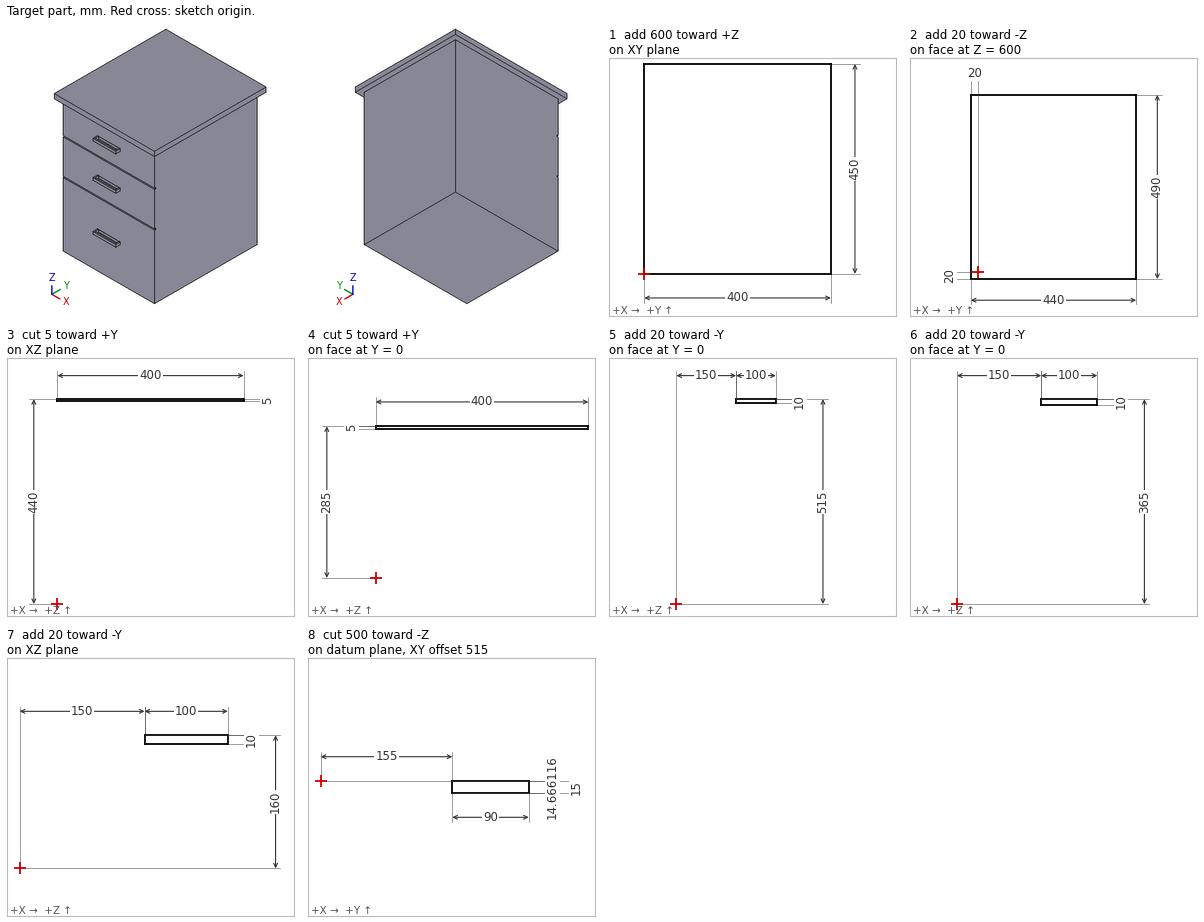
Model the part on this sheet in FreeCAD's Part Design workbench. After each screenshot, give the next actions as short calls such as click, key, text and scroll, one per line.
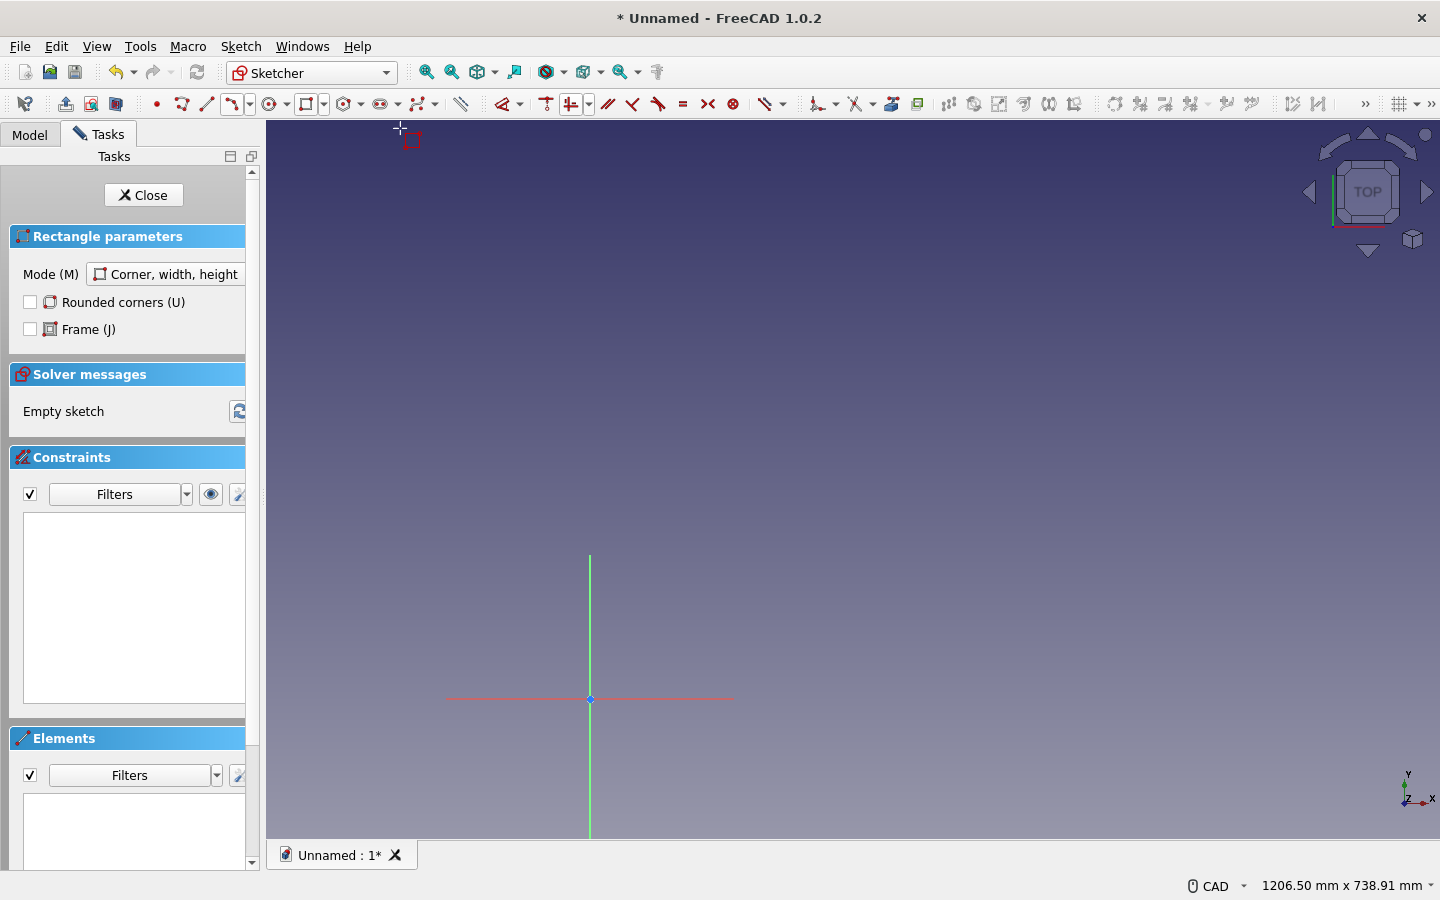
click(590, 699)
move(980, 262)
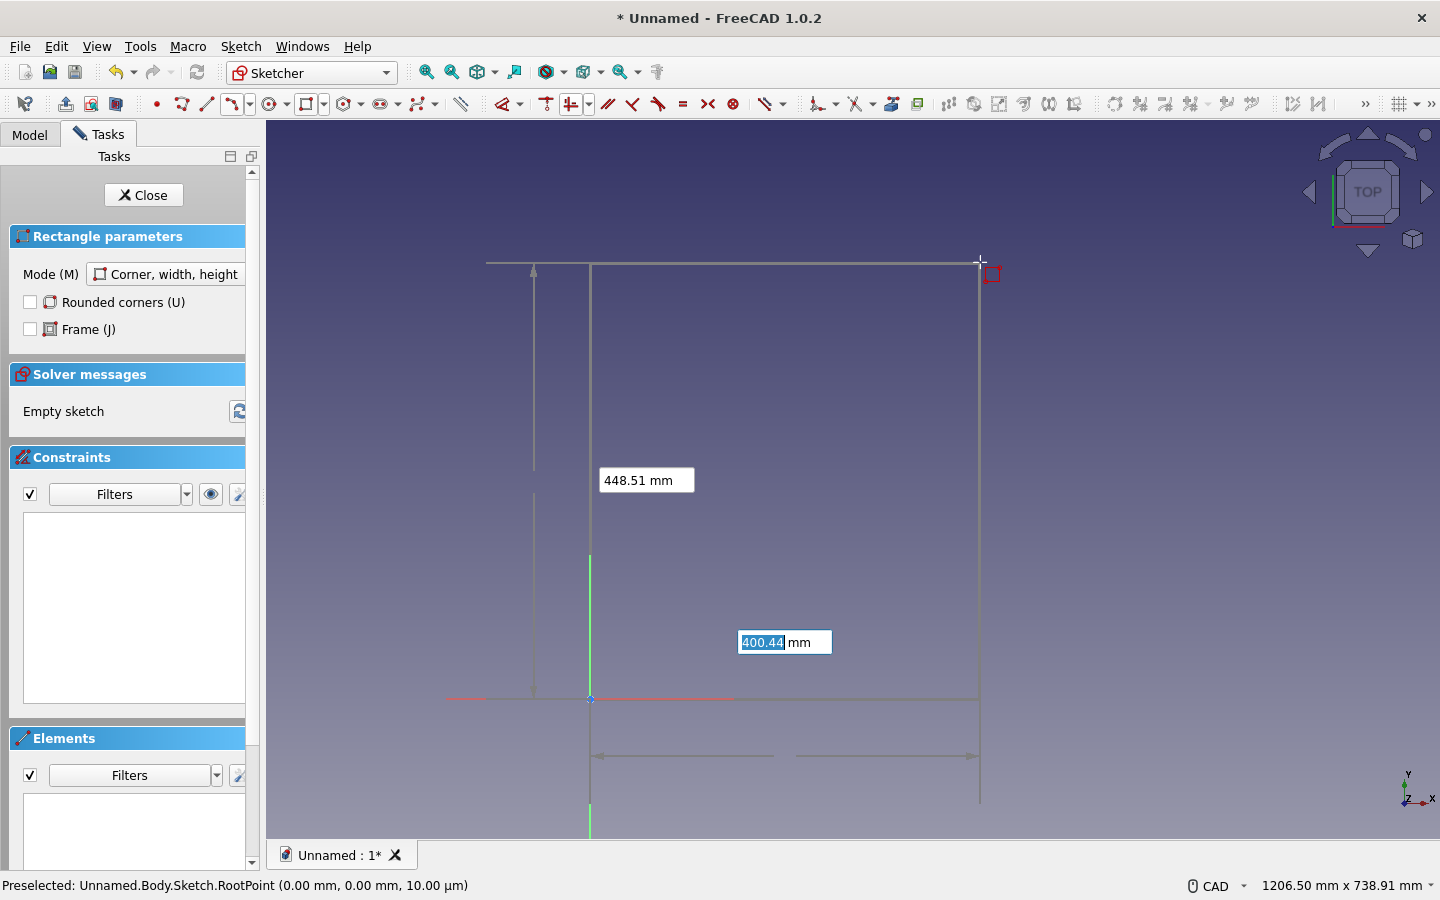
text(400)
key(Tab)
text(450)
key(Return)
key(Escape)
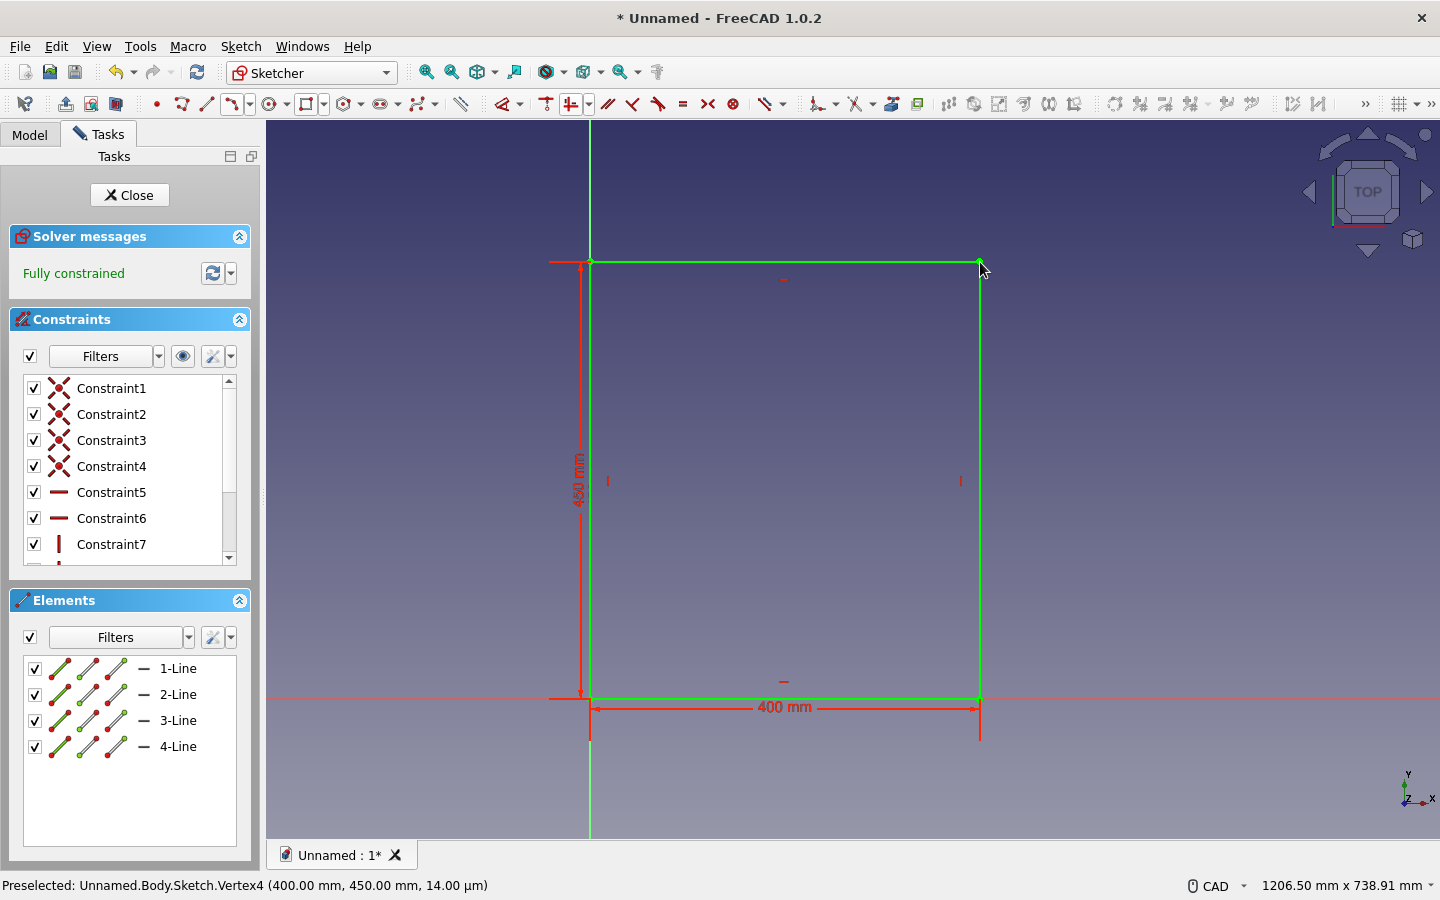
click(130, 195)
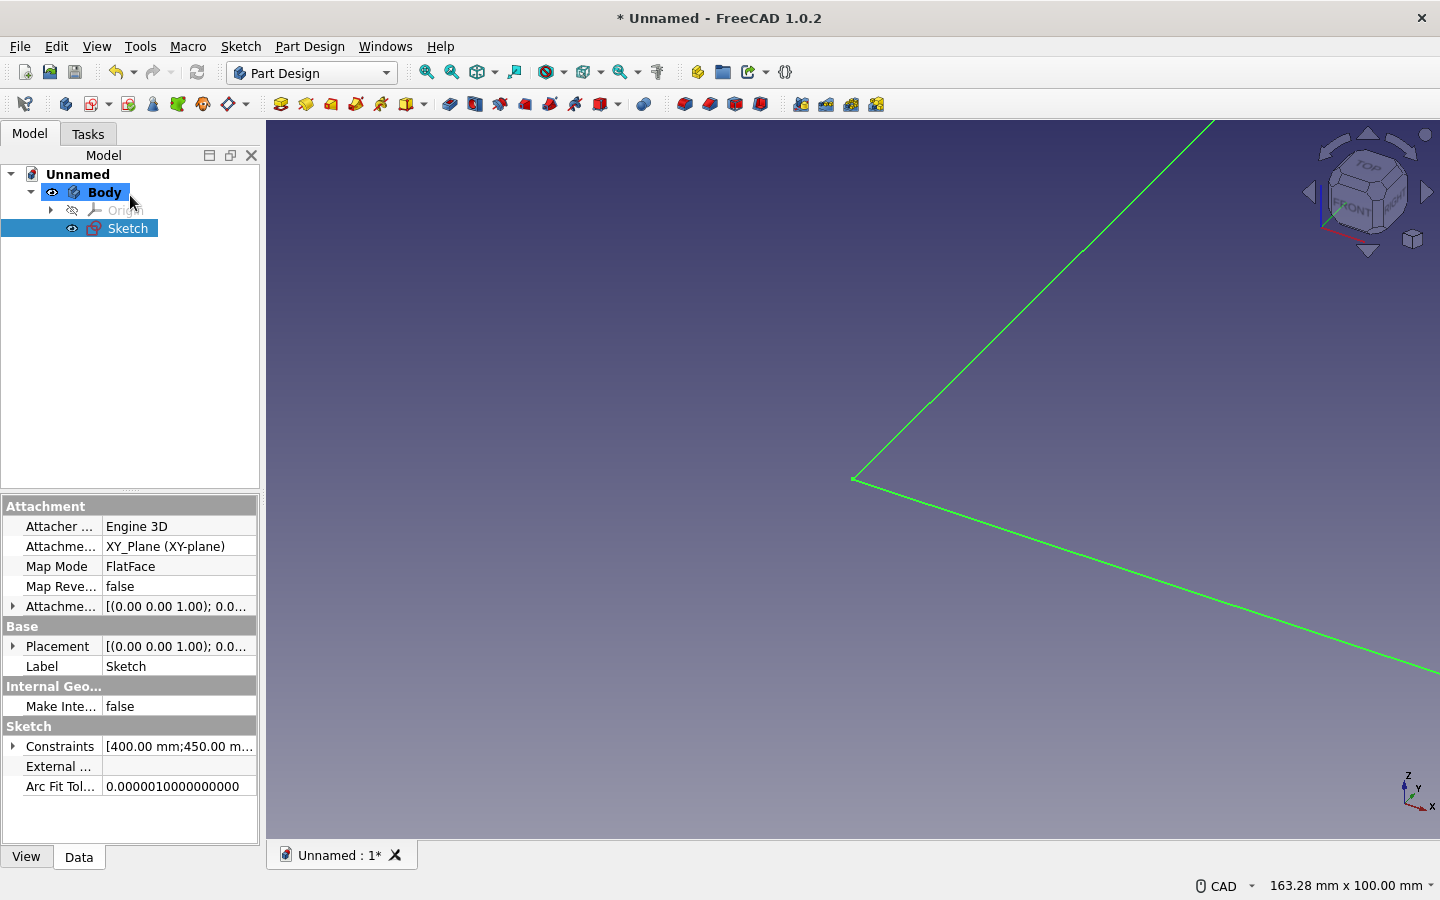
click(281, 104)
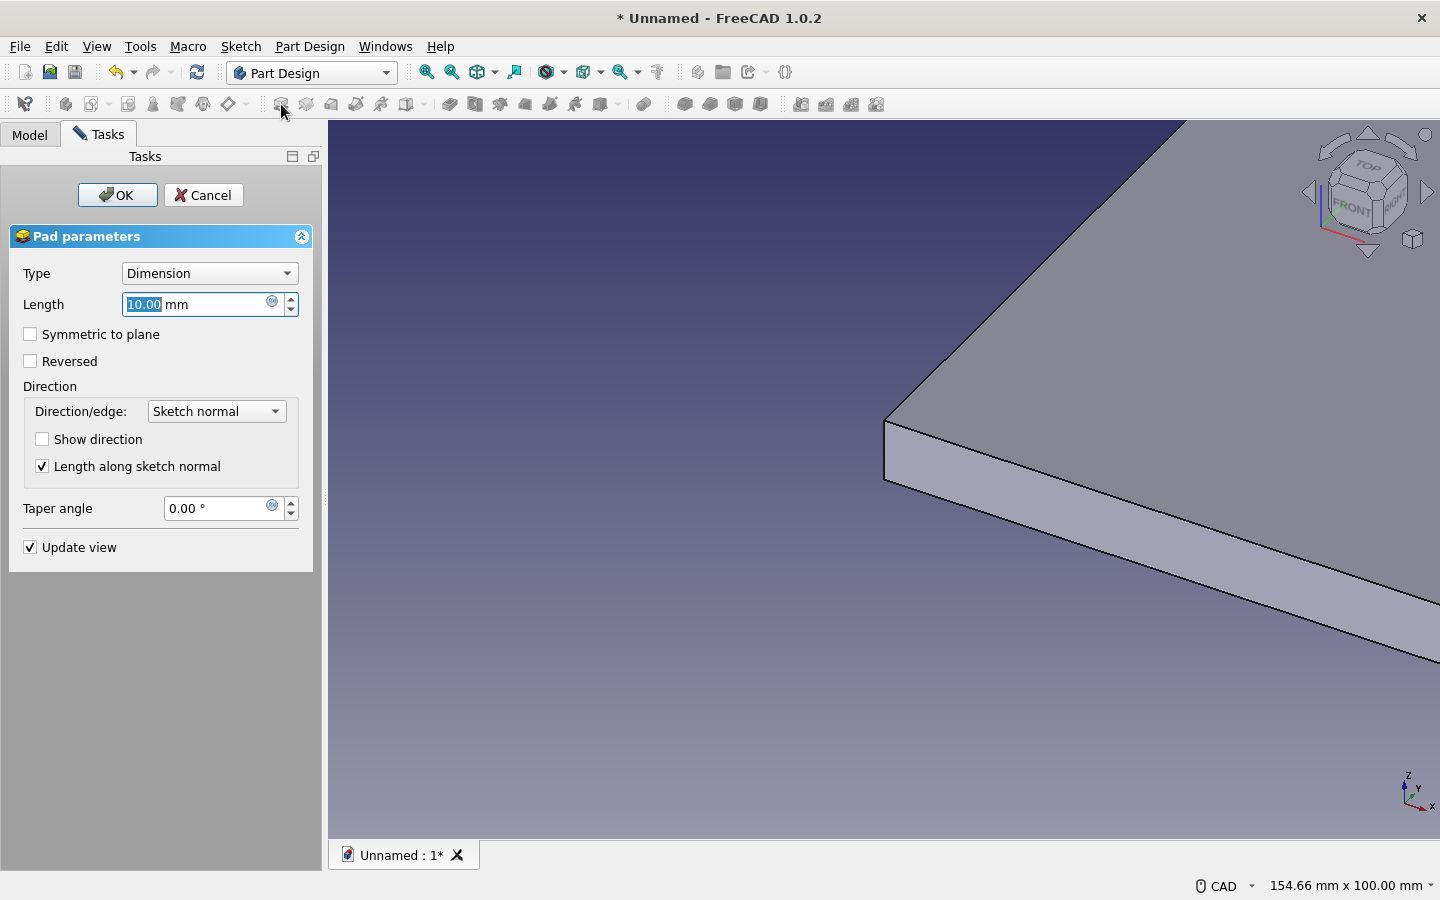
text(600)
key(Tab)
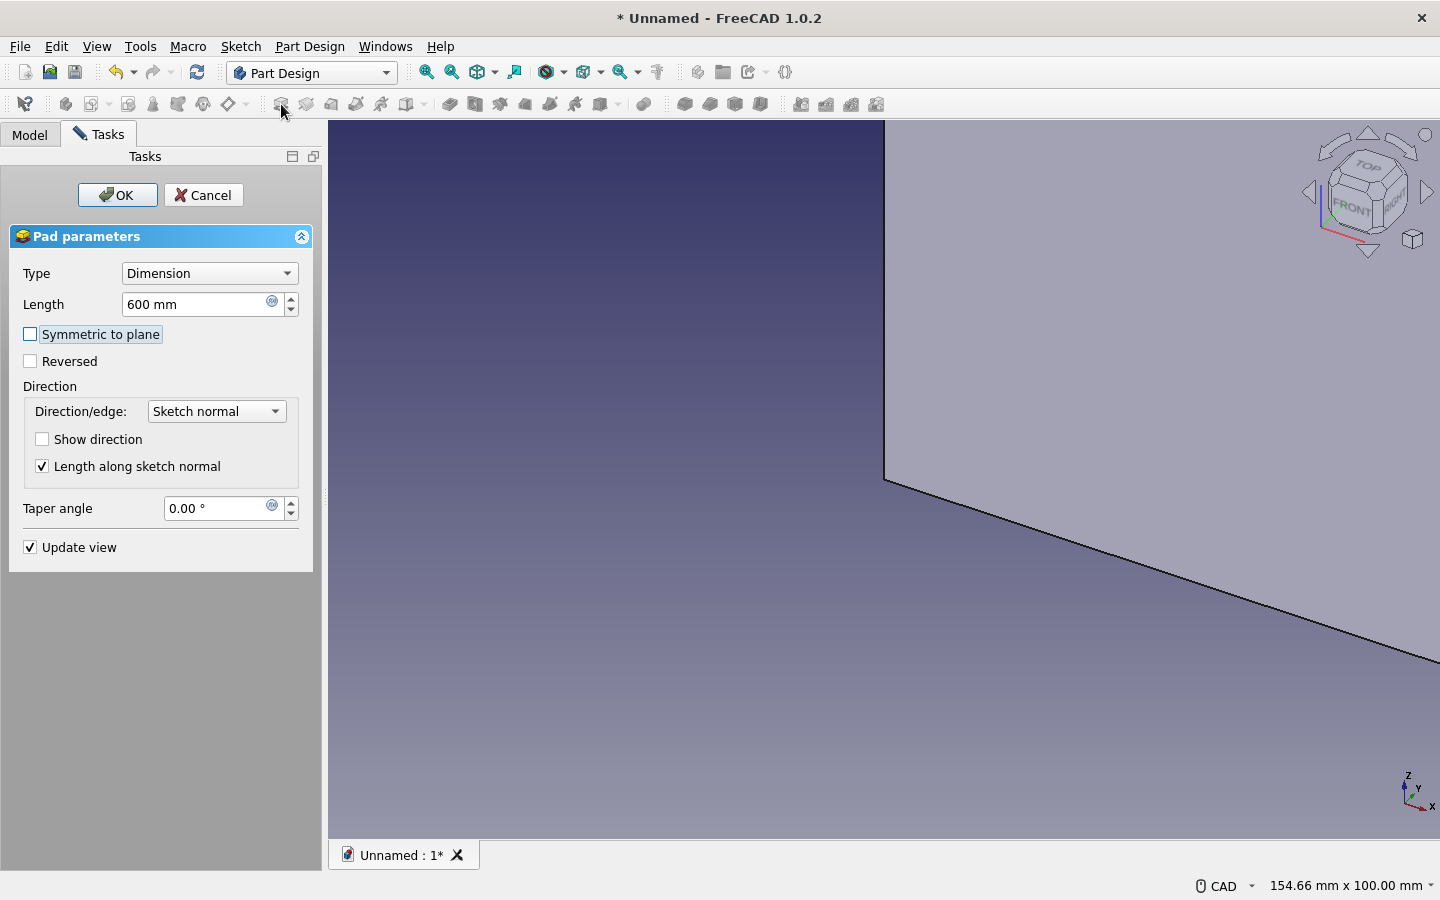
click(118, 195)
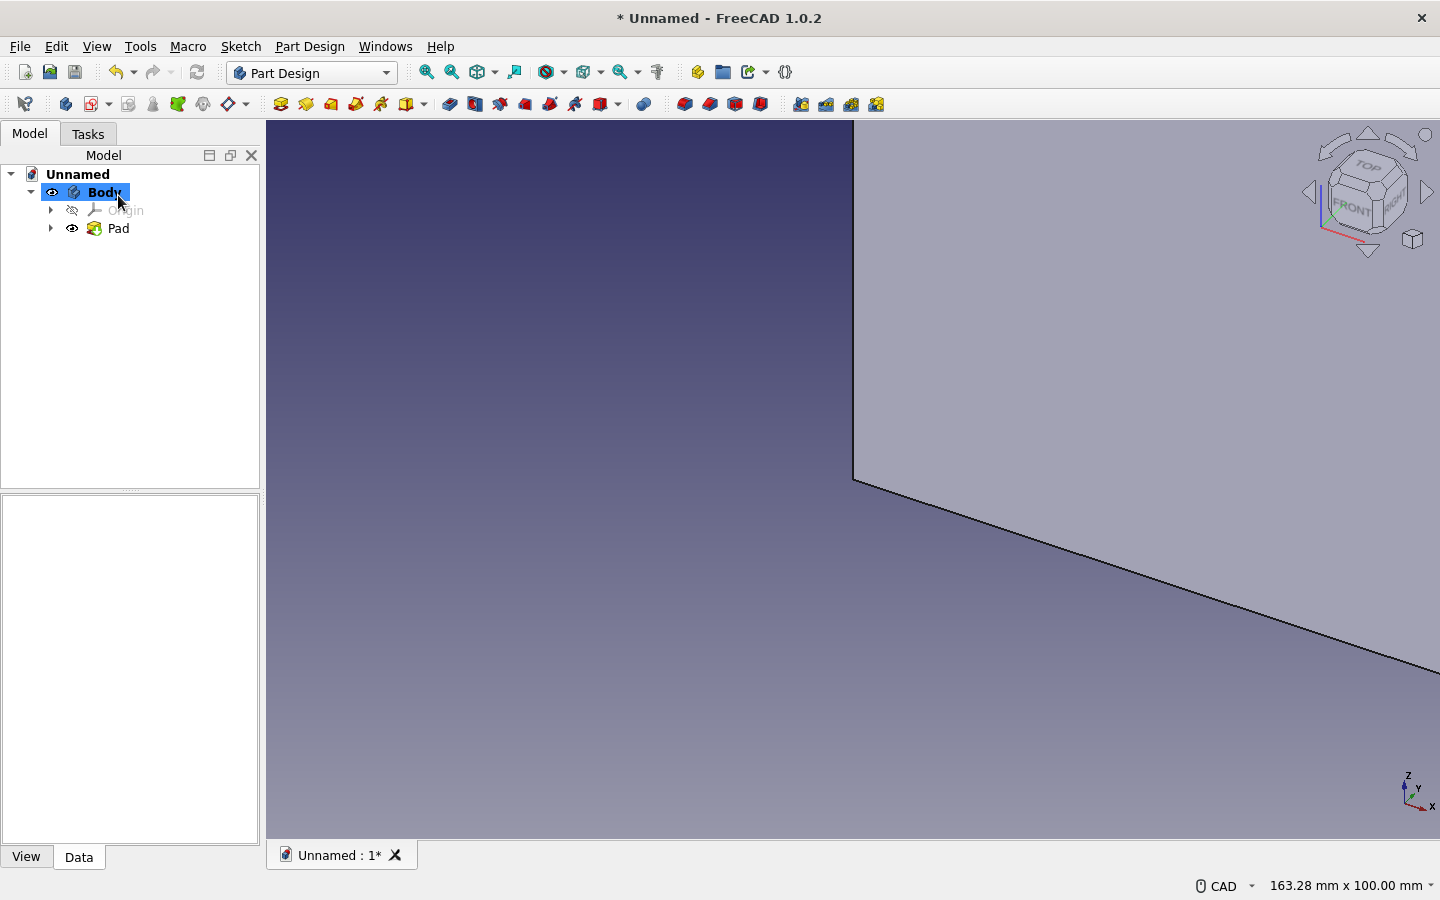
click(427, 72)